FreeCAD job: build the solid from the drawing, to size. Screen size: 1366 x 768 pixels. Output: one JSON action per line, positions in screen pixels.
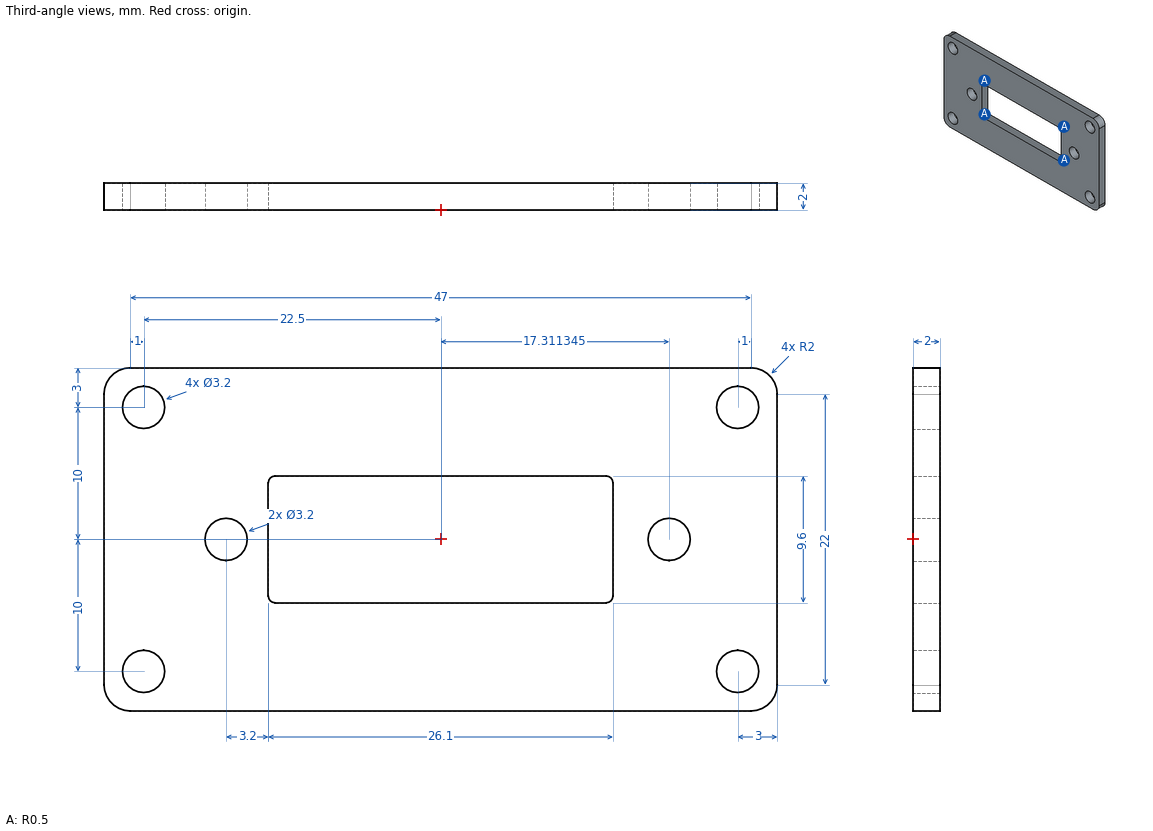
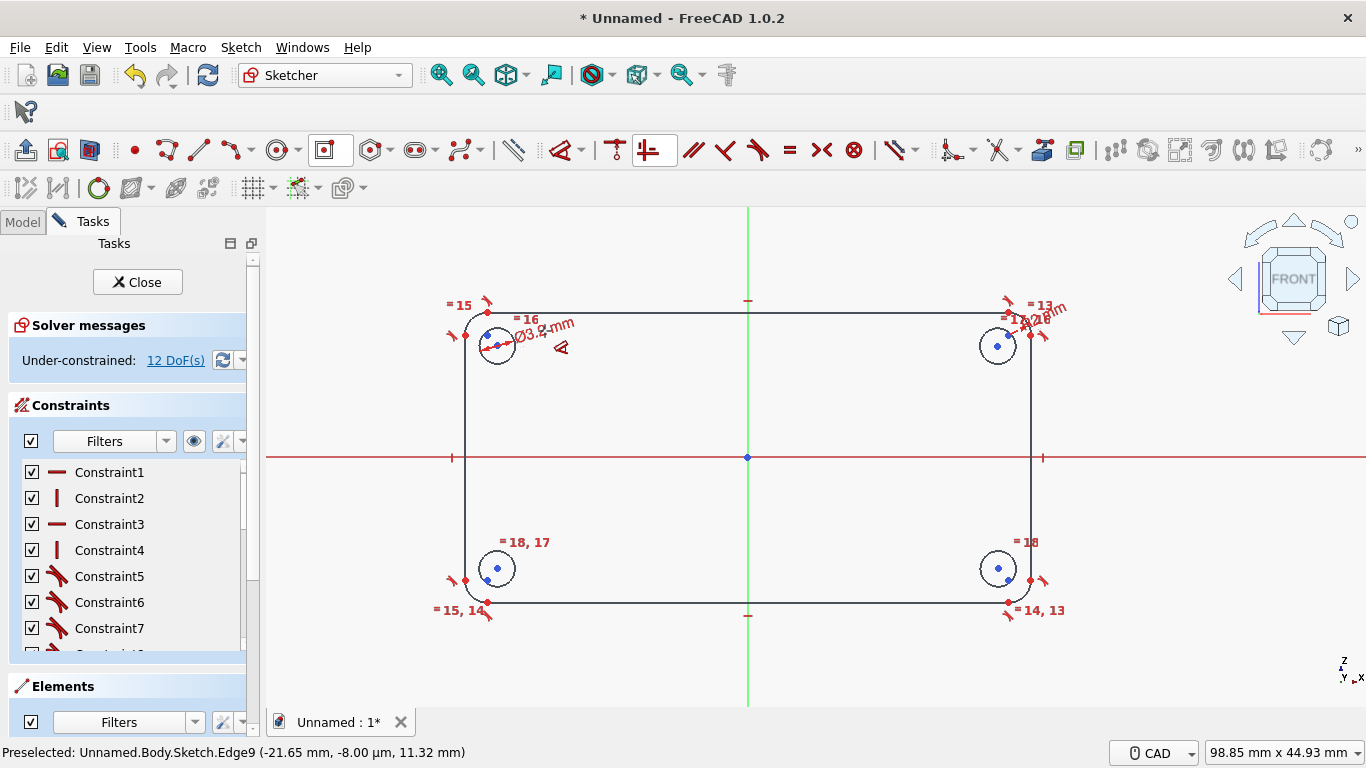
{"action": "left_click", "coordinate": [644, 313]}
{"action": "left_click", "coordinate": [628, 279]}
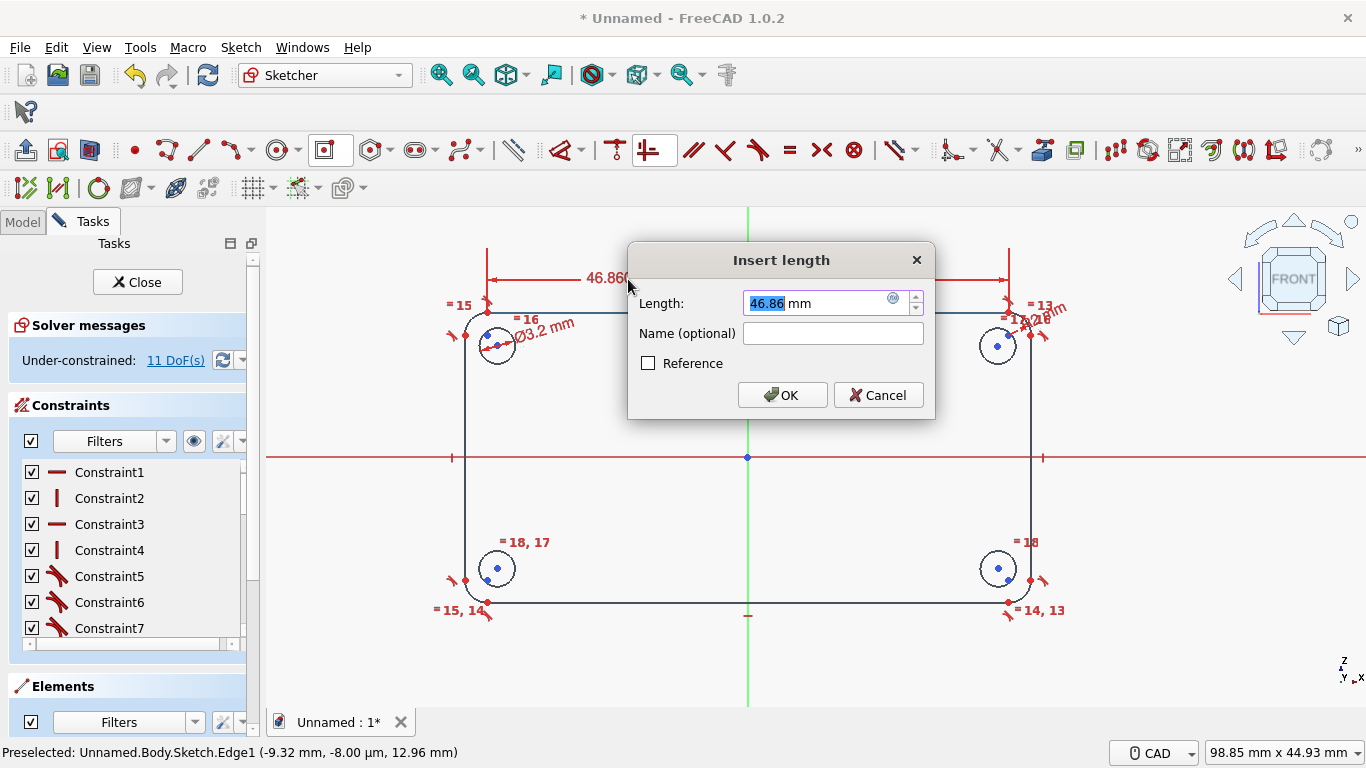
{"action": "type", "text": "47"}
{"action": "key", "text": "Return"}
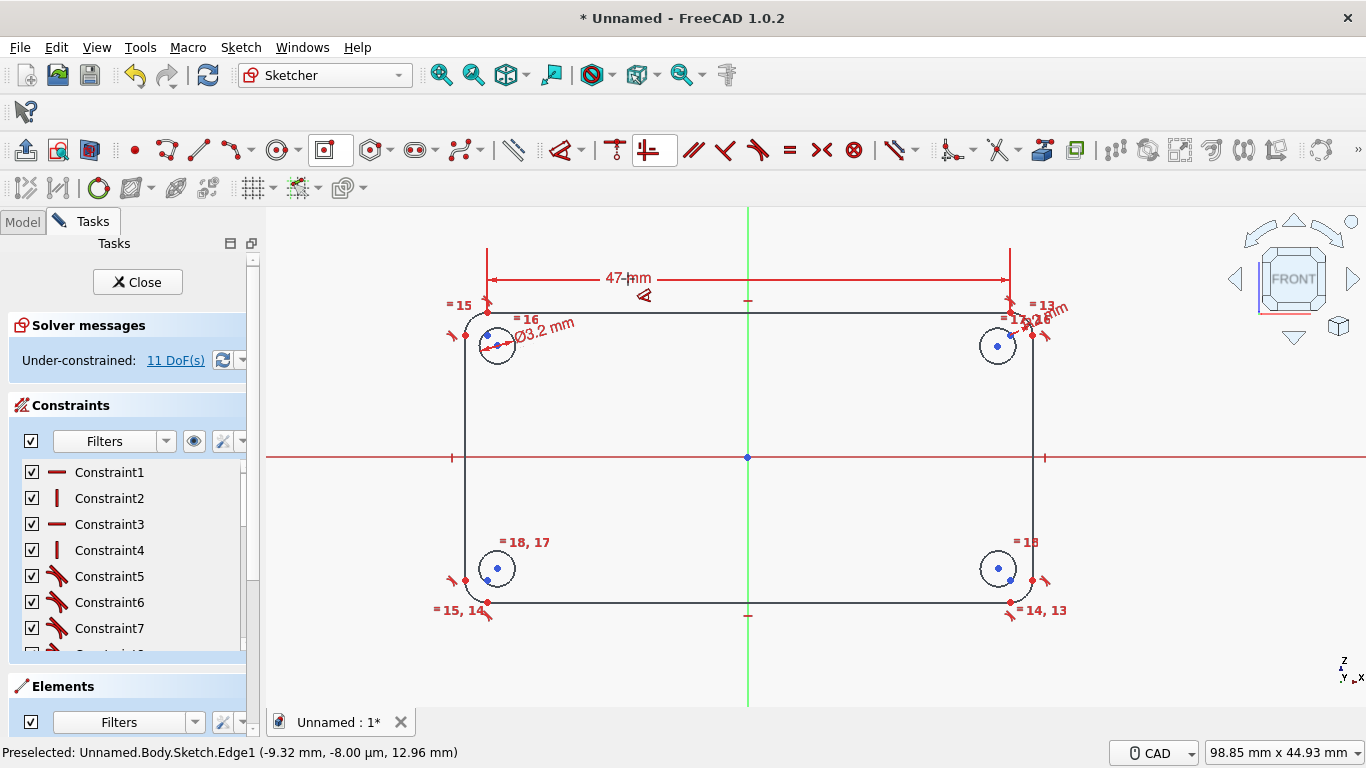
{"action": "left_click", "coordinate": [1033, 409]}
{"action": "left_click", "coordinate": [1067, 401]}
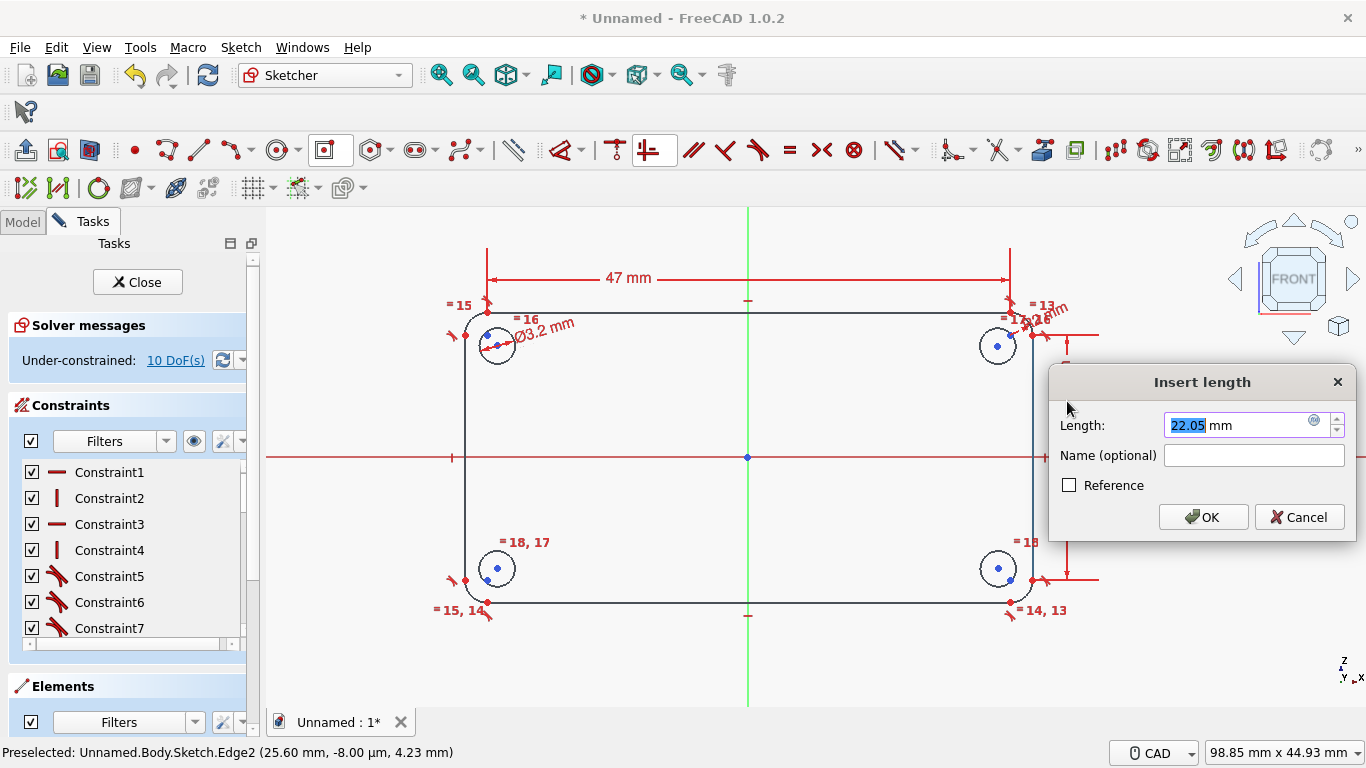
{"action": "type", "text": "22"}
{"action": "key", "text": "Return"}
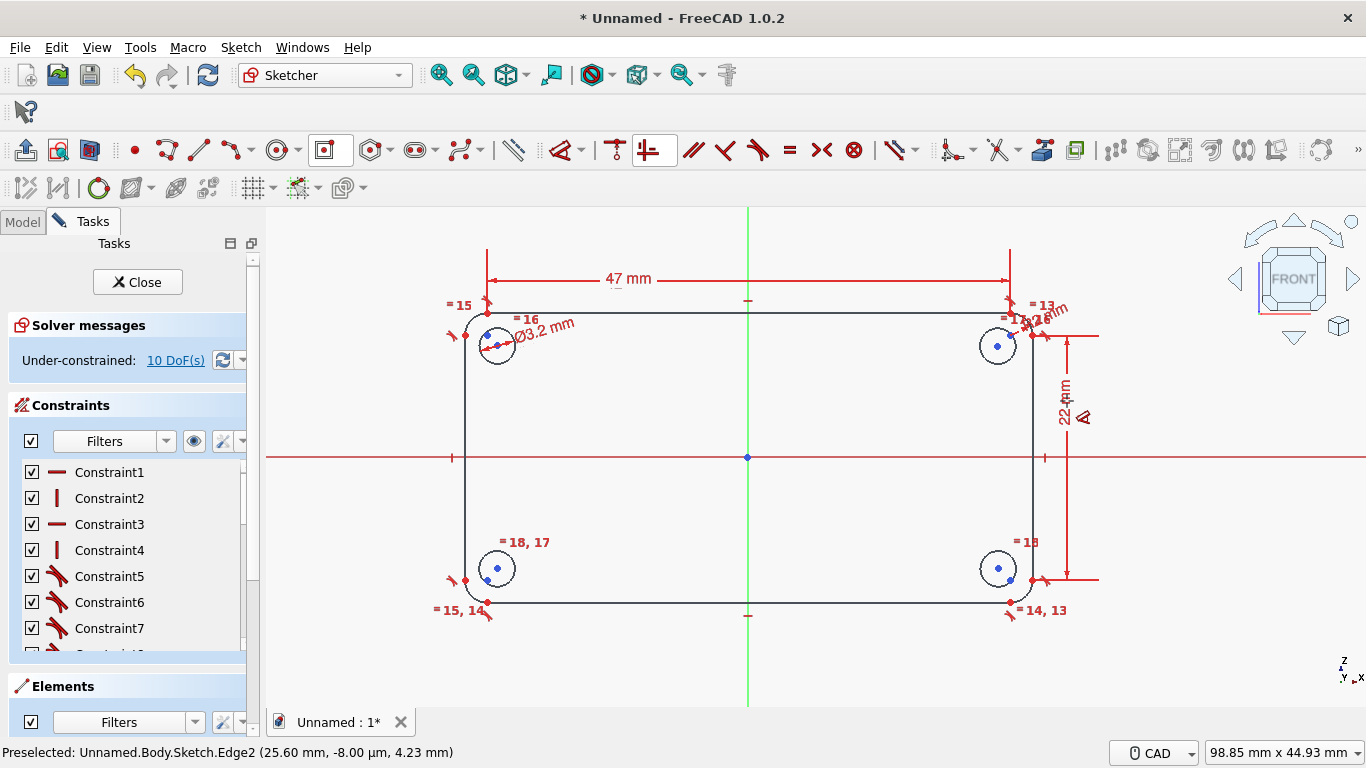
{"action": "left_click", "coordinate": [497, 346]}
{"action": "left_click", "coordinate": [782, 402]}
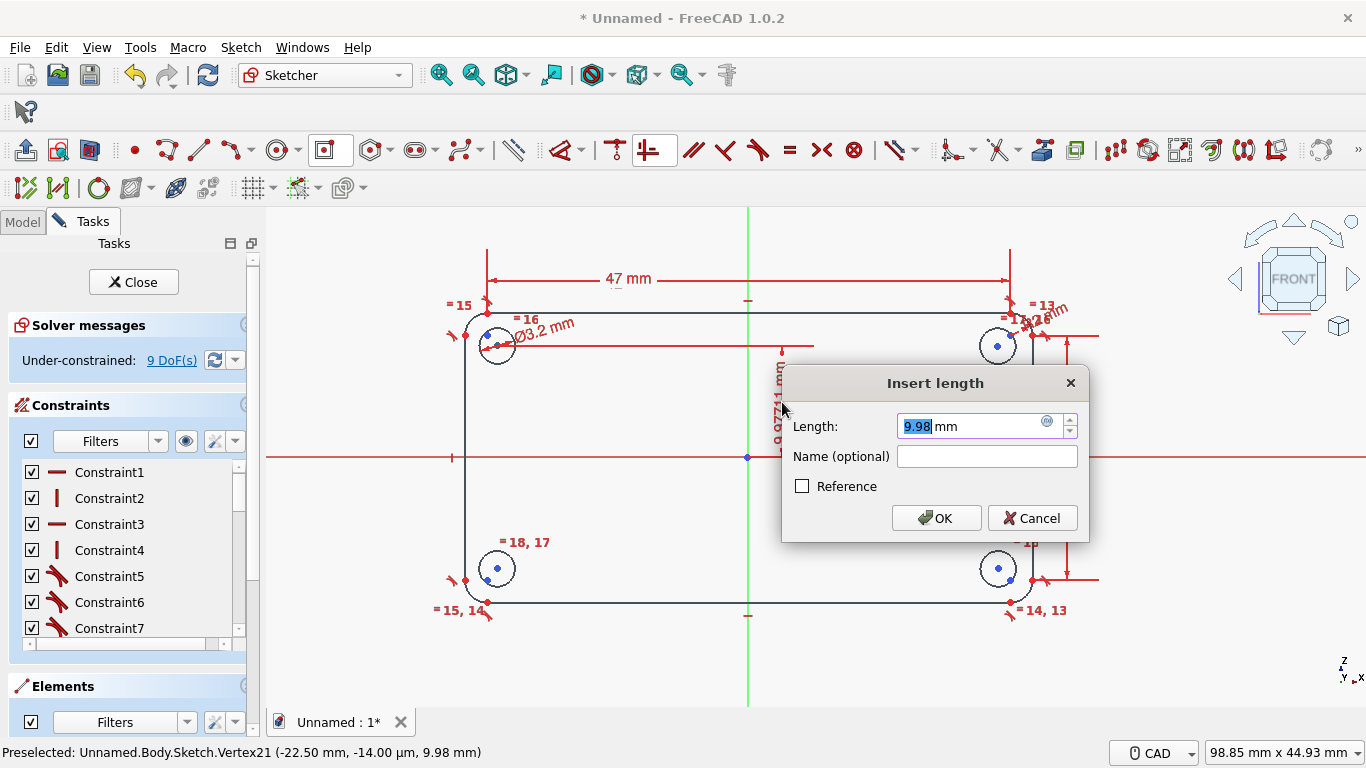
{"action": "type", "text": "10"}
{"action": "key", "text": "Return"}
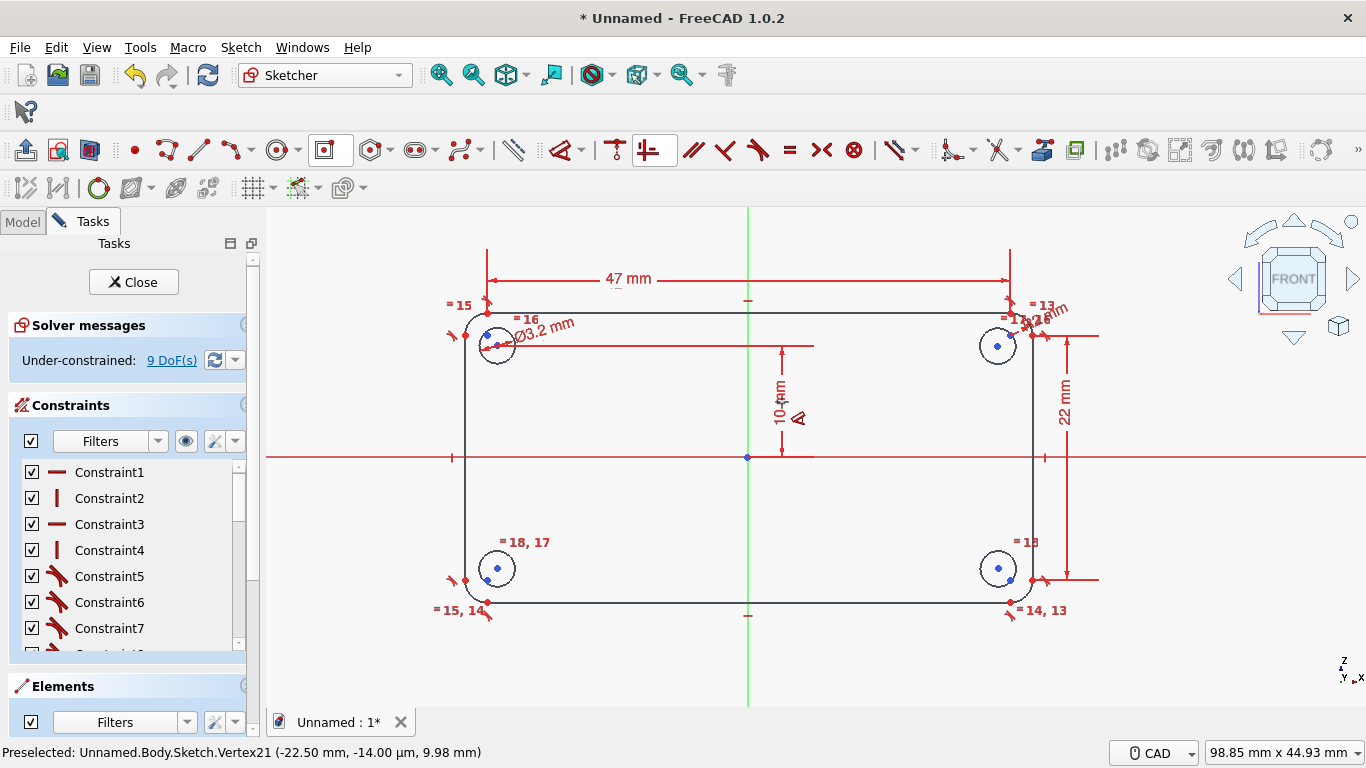
{"action": "left_click", "coordinate": [998, 346]}
{"action": "left_click", "coordinate": [714, 376]}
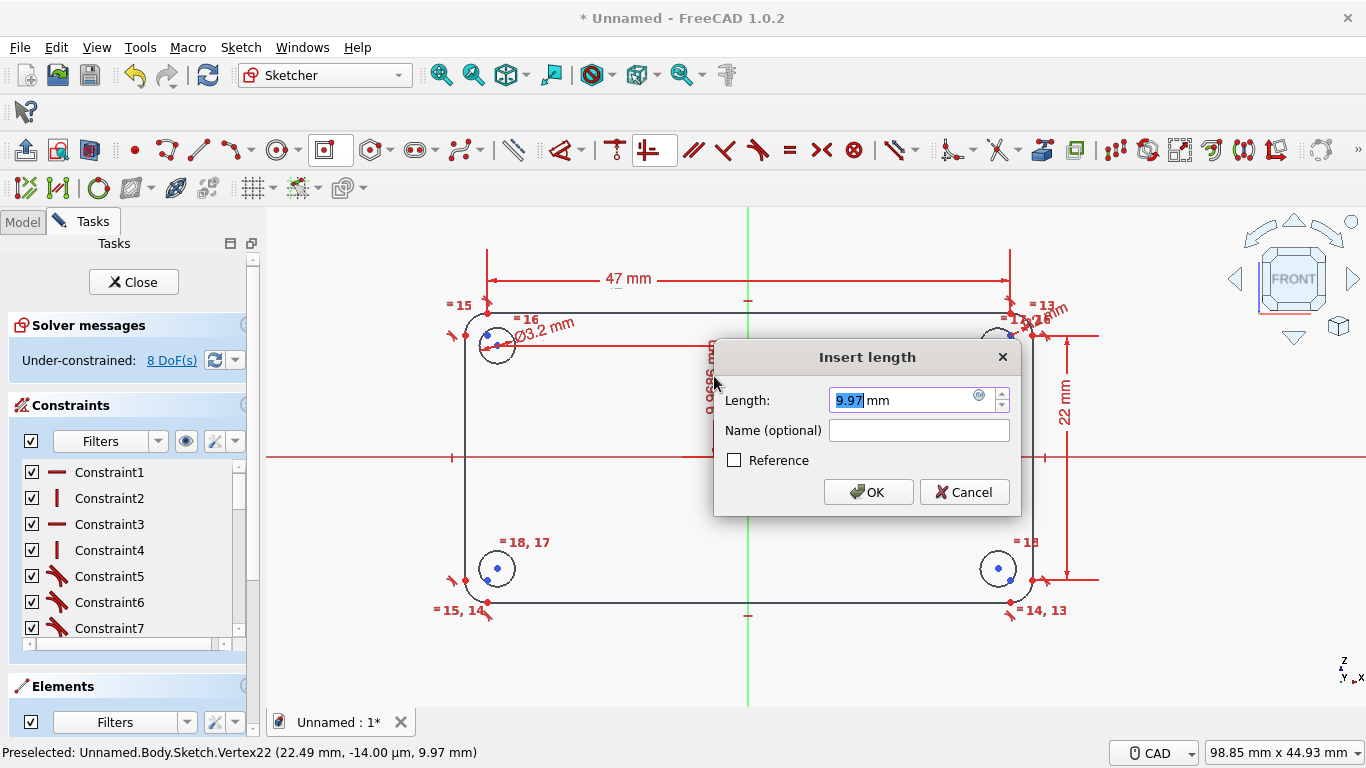
{"action": "type", "text": "10"}
{"action": "key", "text": "Return"}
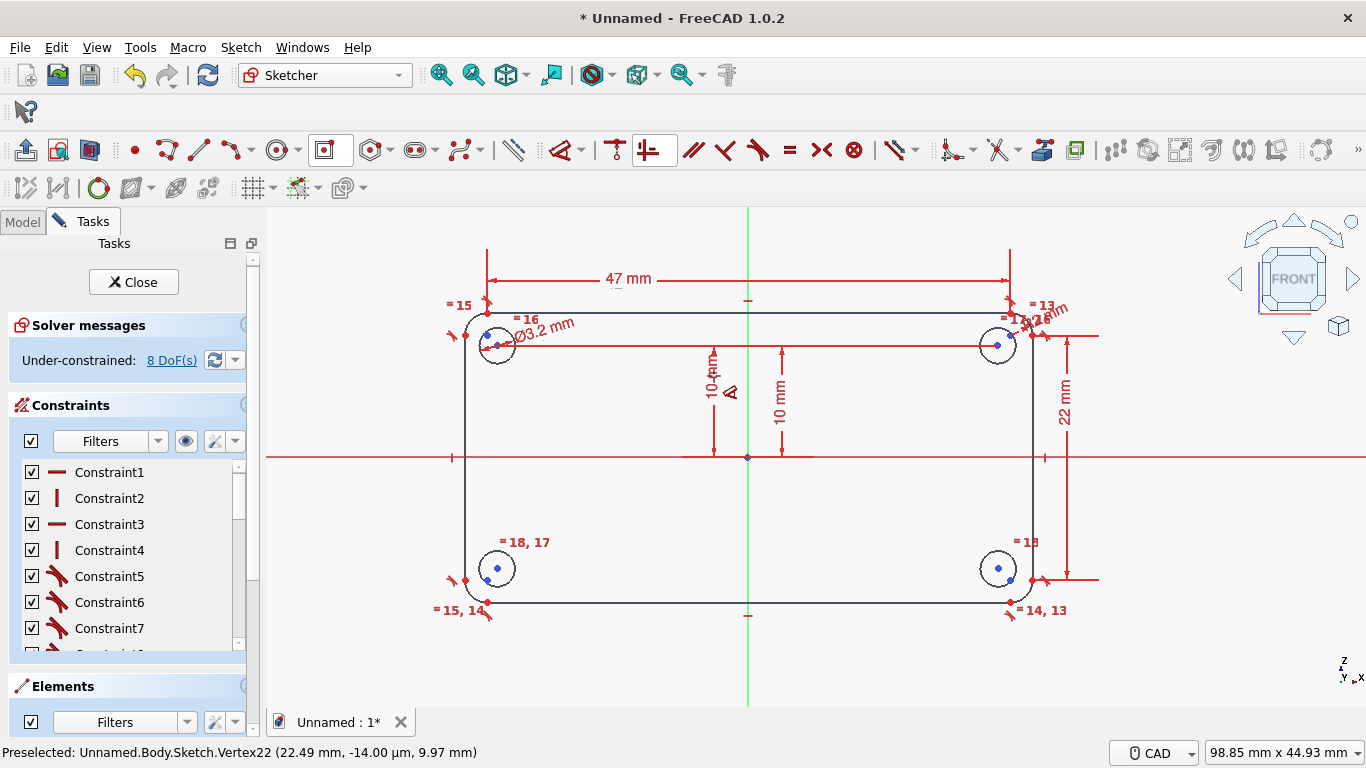
{"action": "left_click", "coordinate": [497, 569]}
{"action": "left_click", "coordinate": [782, 513]}